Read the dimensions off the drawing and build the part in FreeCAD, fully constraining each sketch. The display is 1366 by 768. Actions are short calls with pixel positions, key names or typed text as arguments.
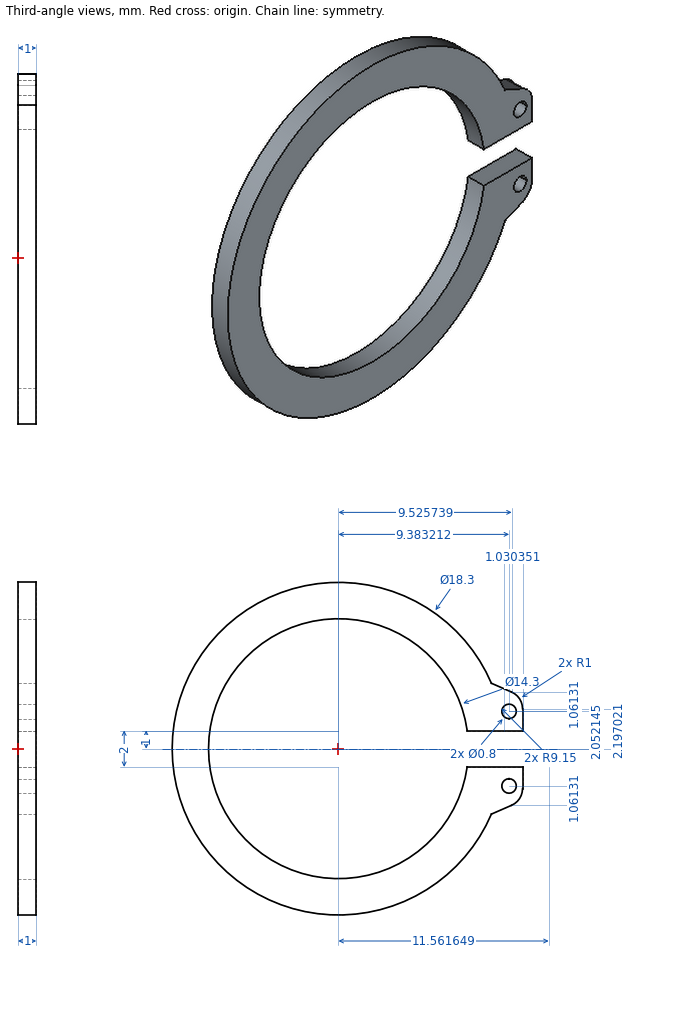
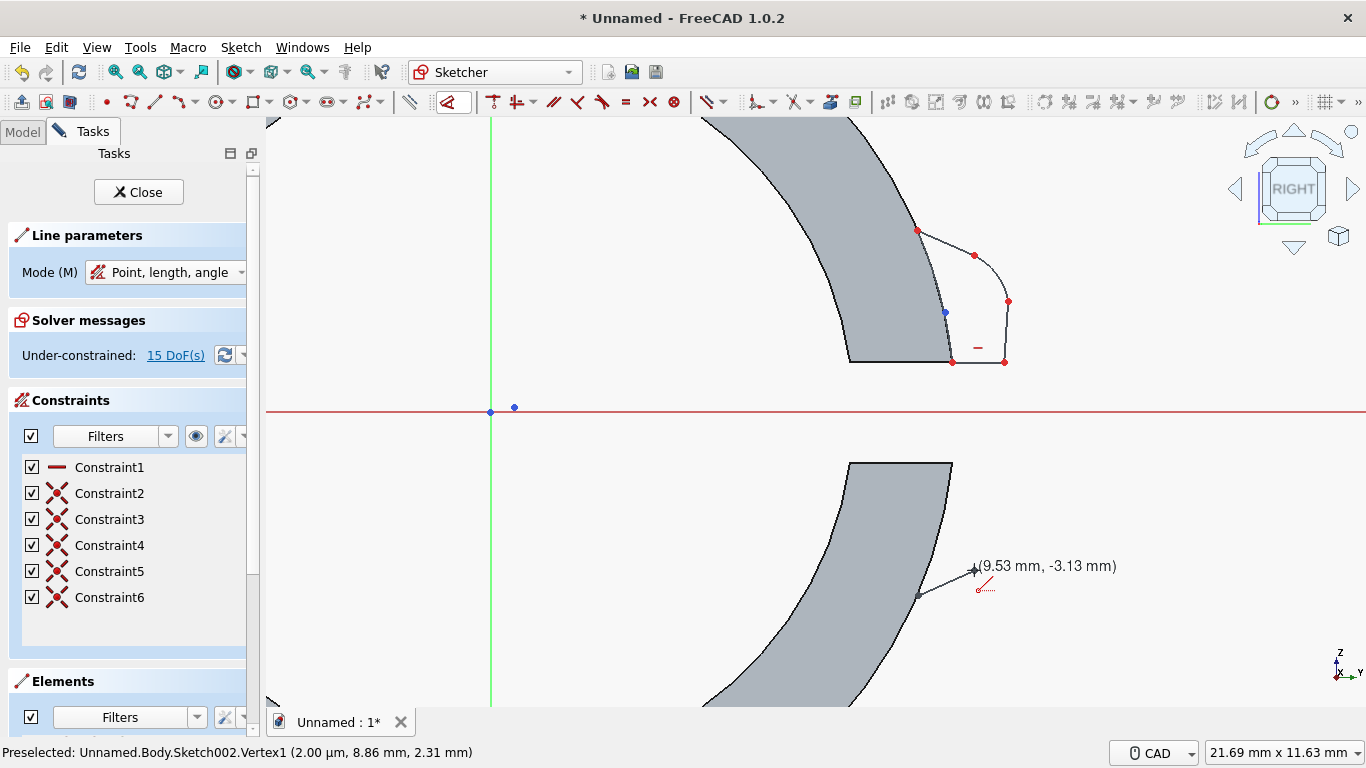
key(g)
key(m)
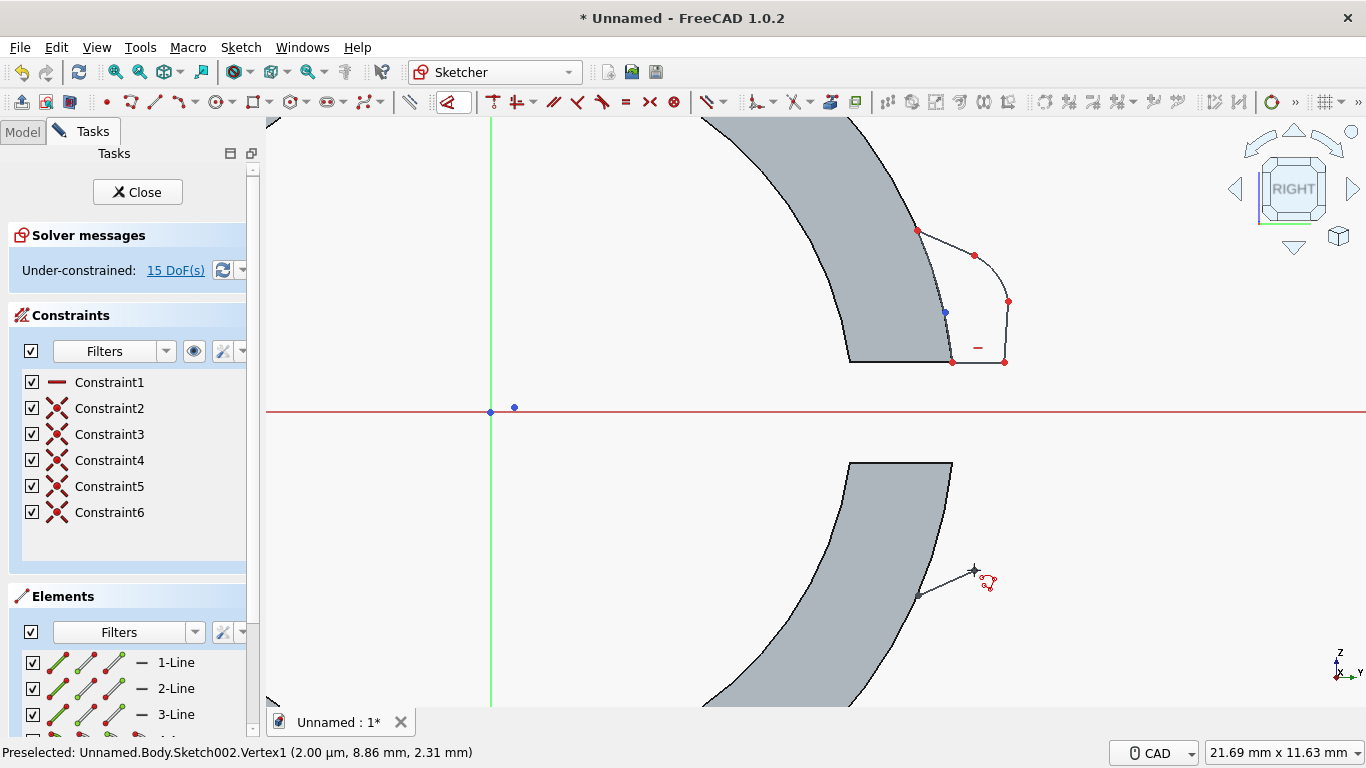
click(1004, 524)
click(1000, 463)
click(952, 463)
right_click(952, 463)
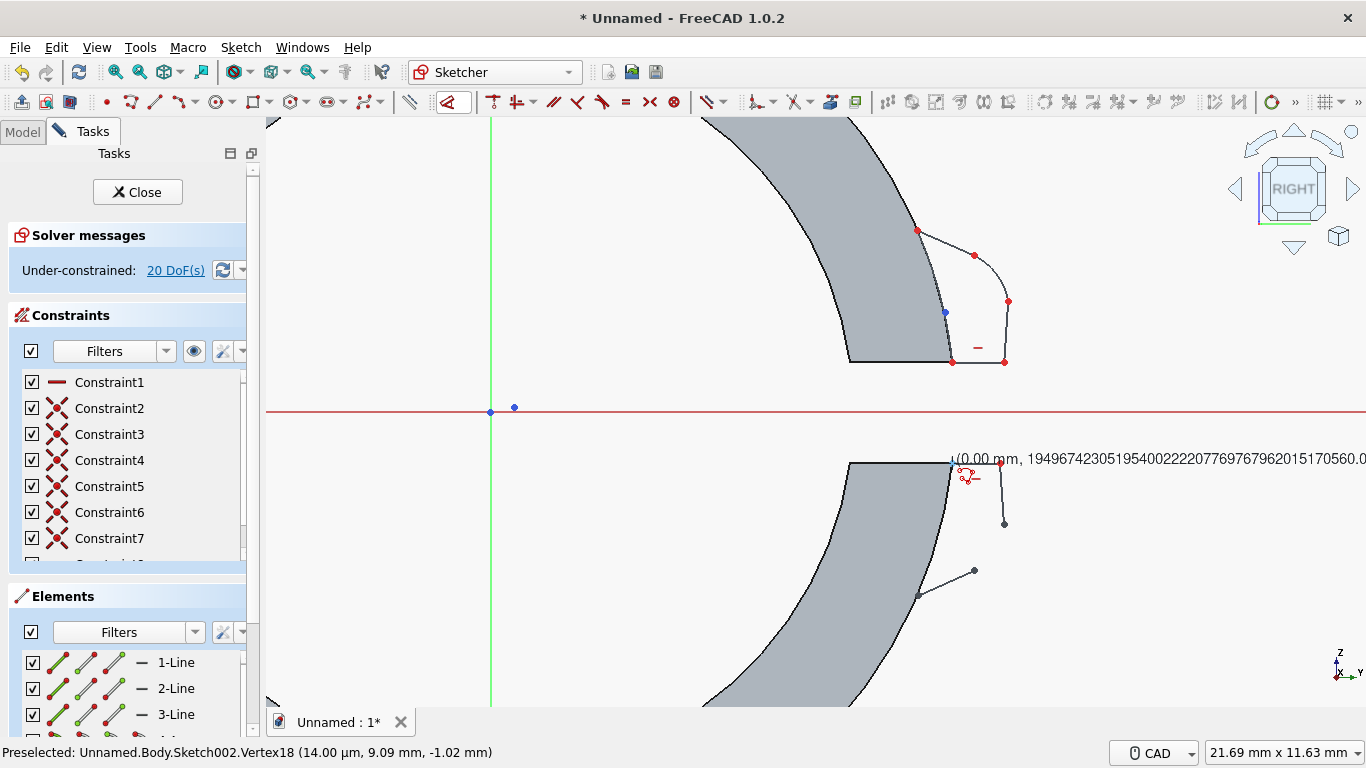
click(180, 102)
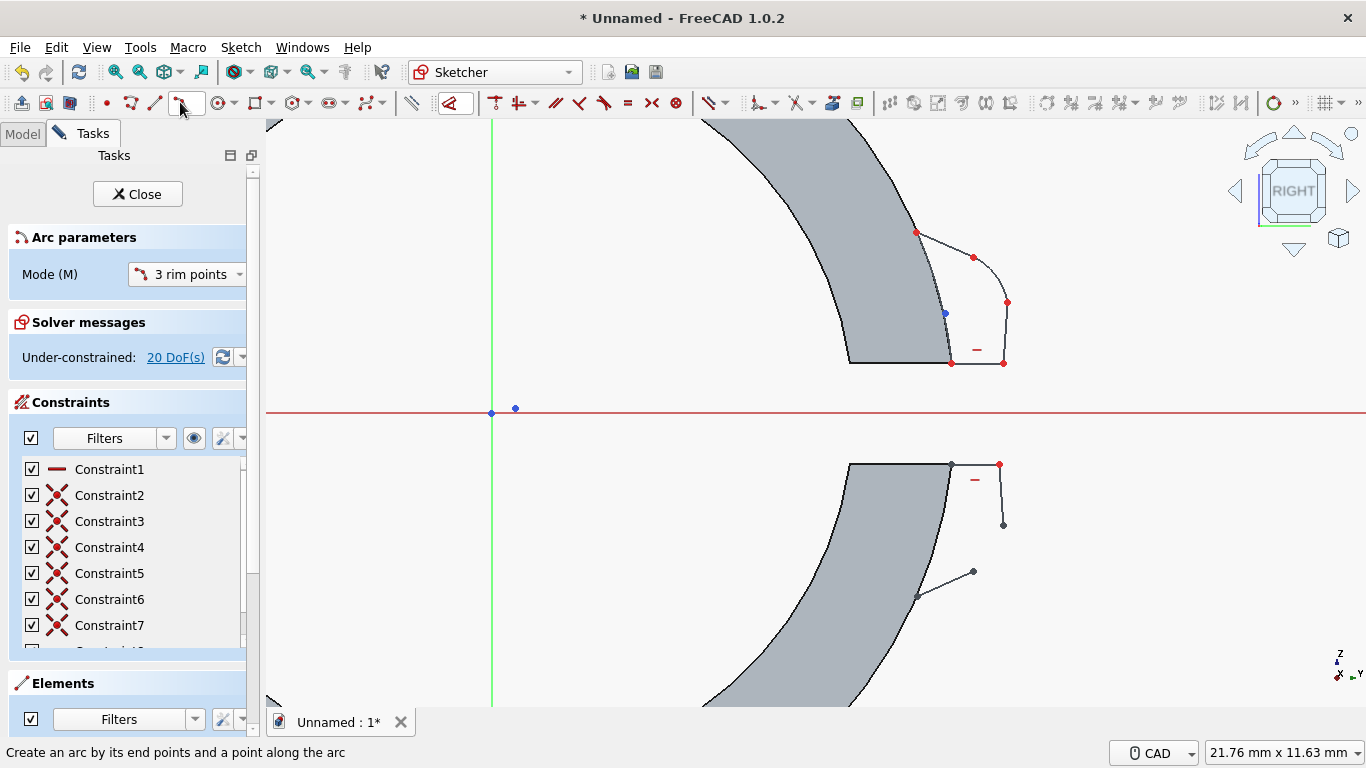
click(973, 571)
click(1003, 526)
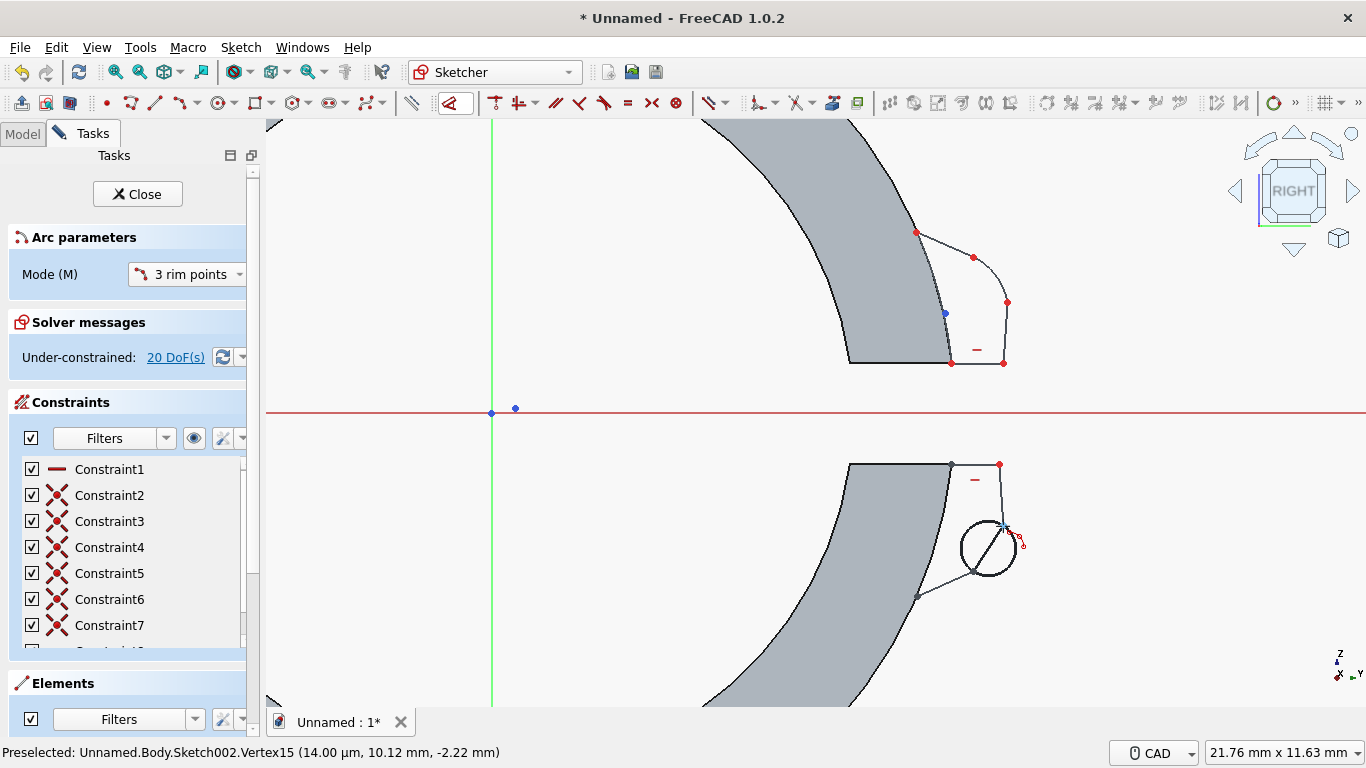
scroll(996, 552, up, 4)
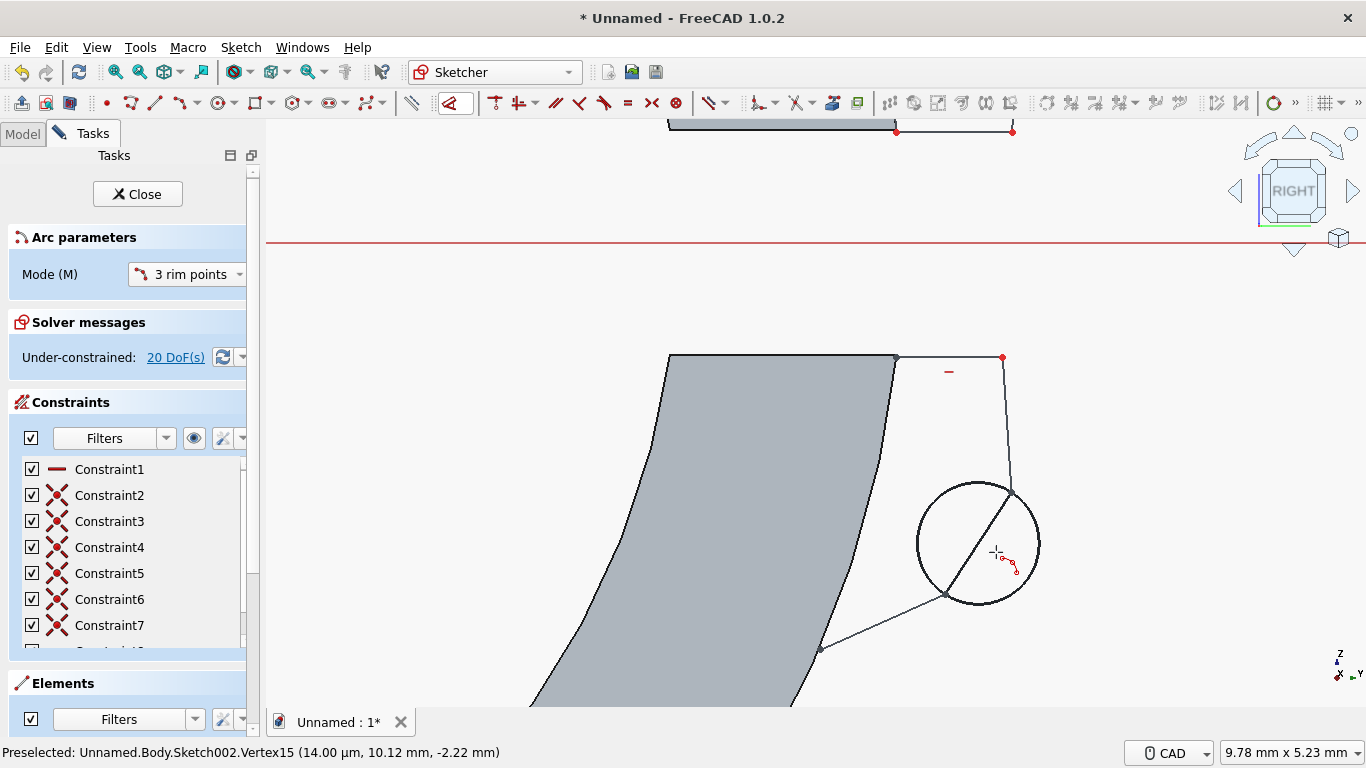
click(994, 551)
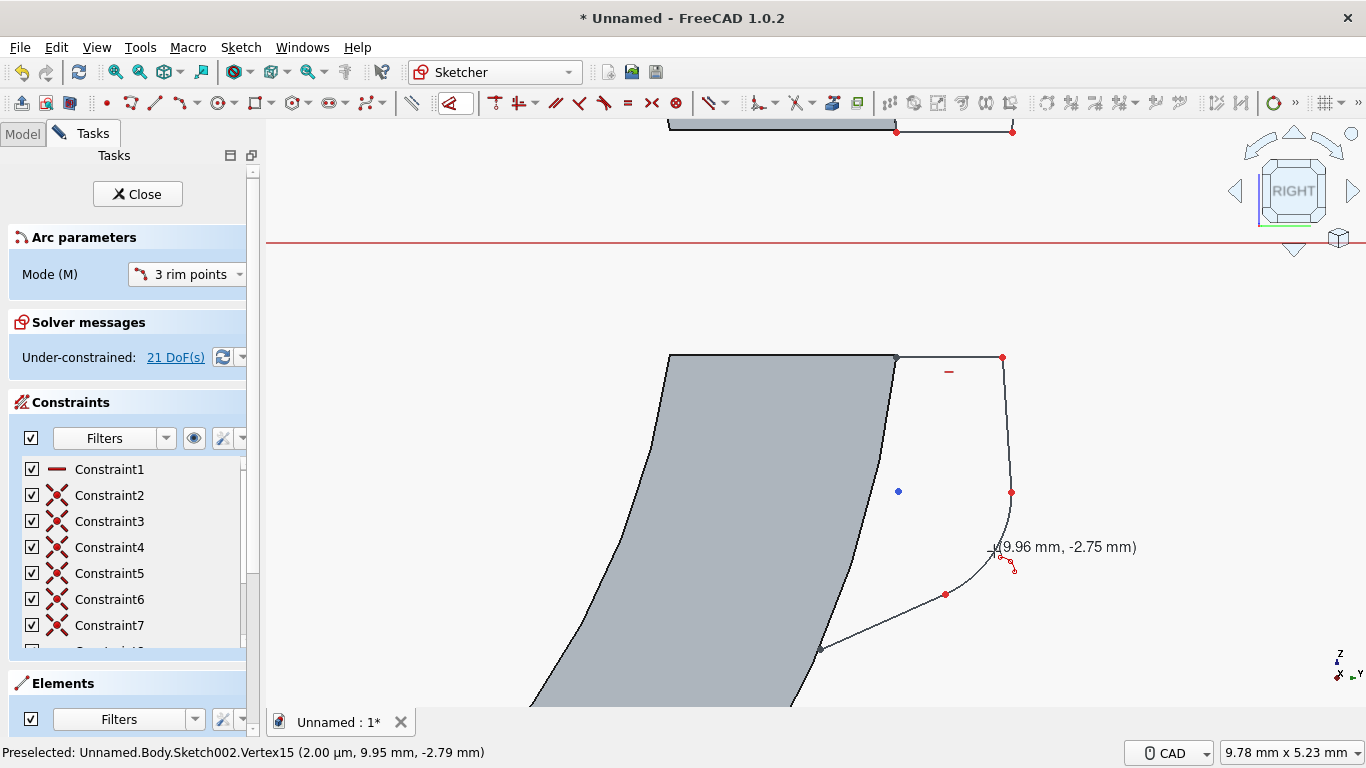
click(896, 357)
click(821, 650)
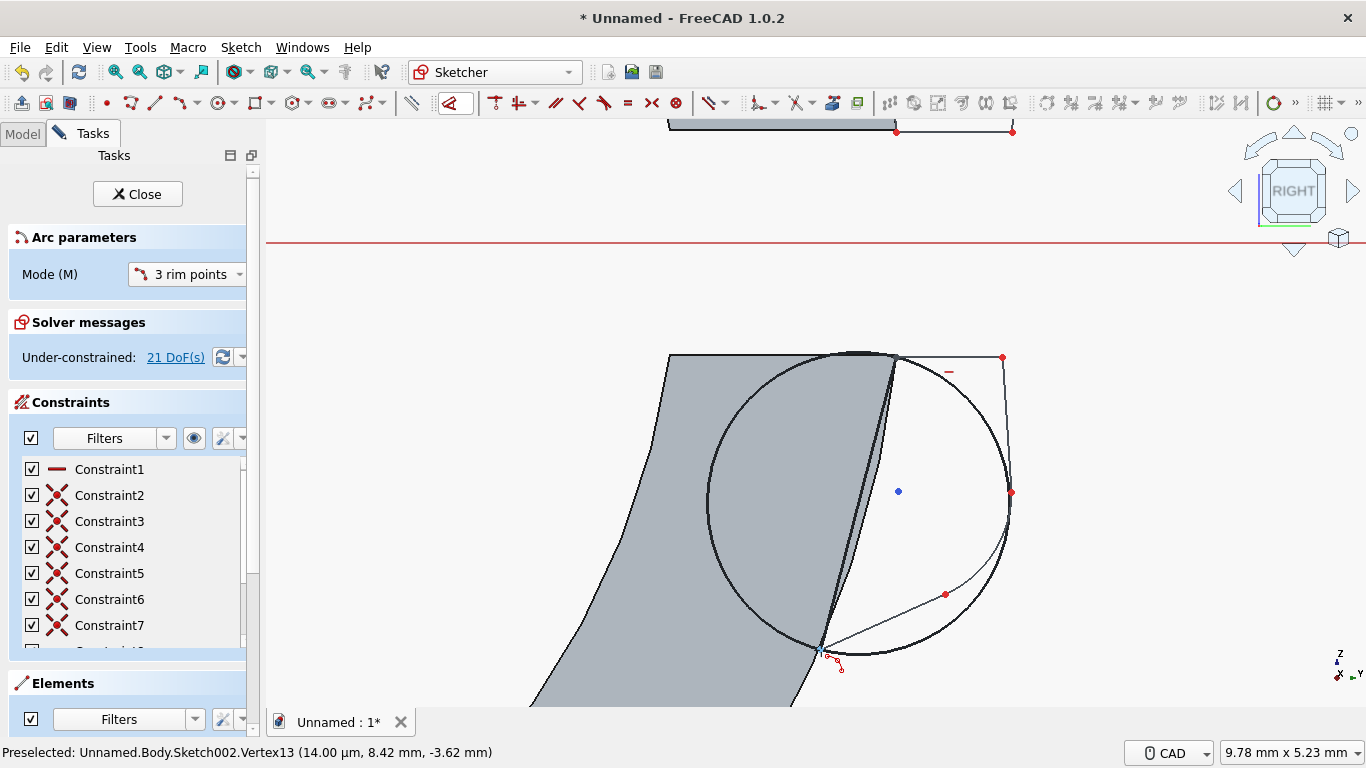
scroll(869, 504, up, 2)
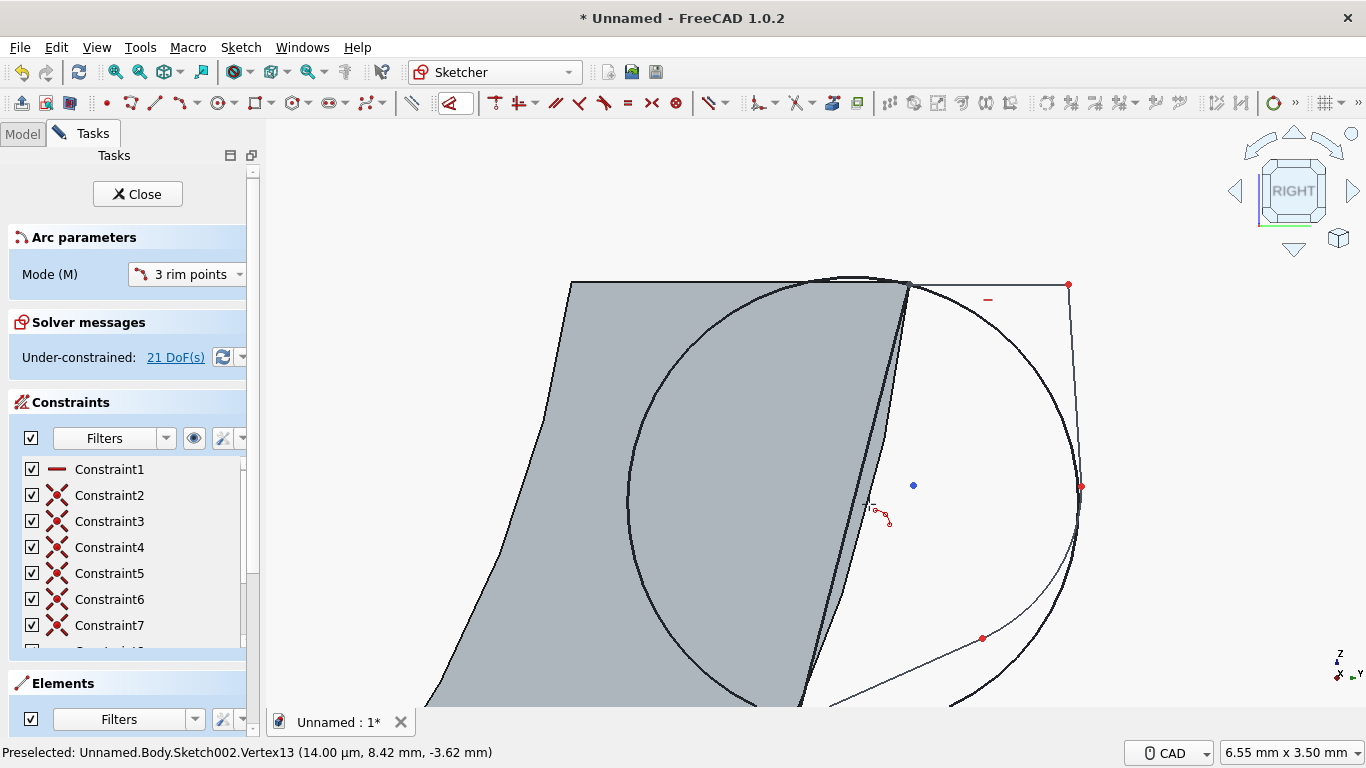
click(869, 504)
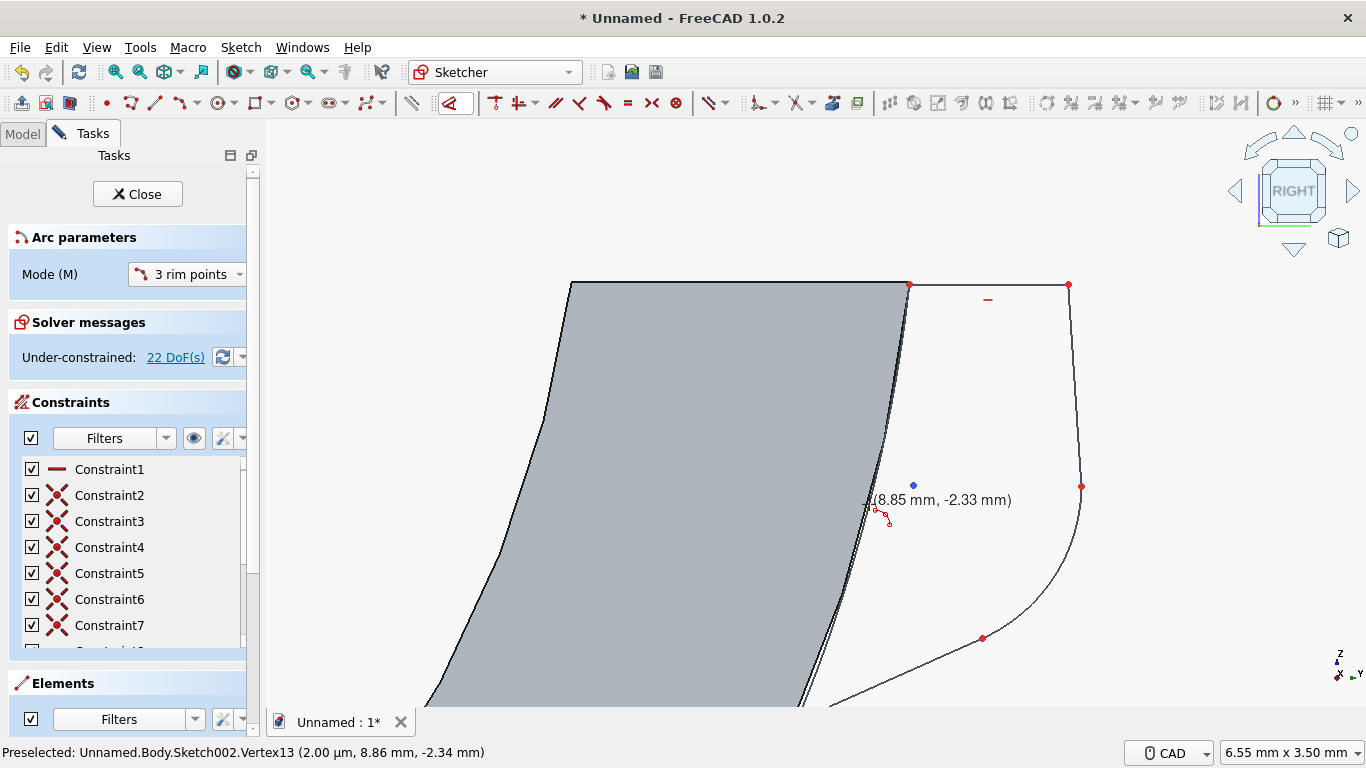
key(g)
key(c)